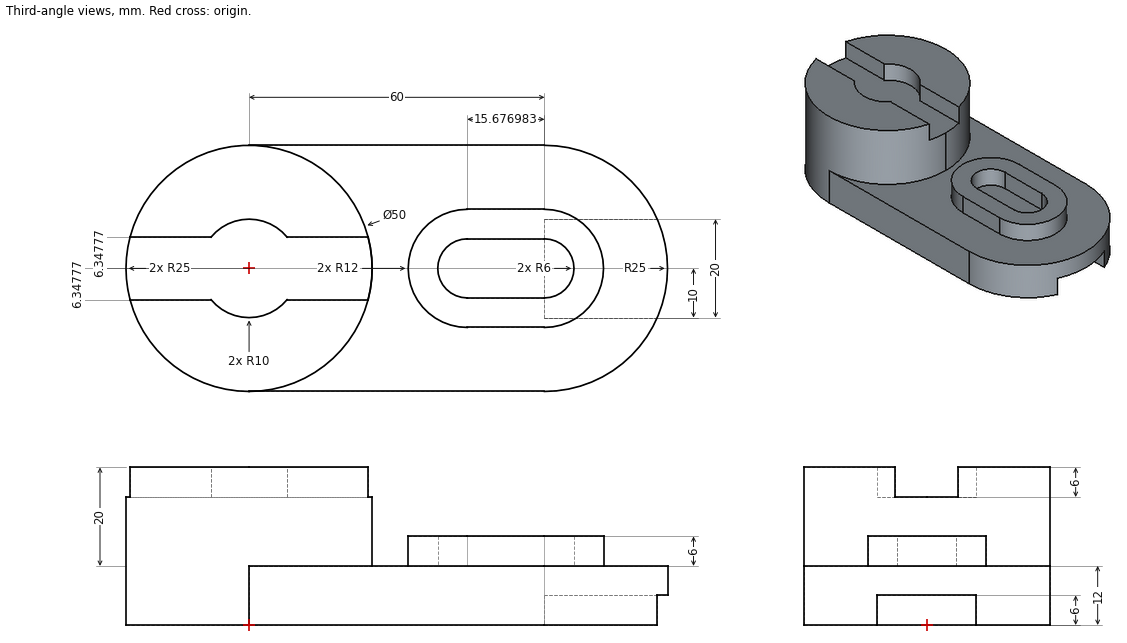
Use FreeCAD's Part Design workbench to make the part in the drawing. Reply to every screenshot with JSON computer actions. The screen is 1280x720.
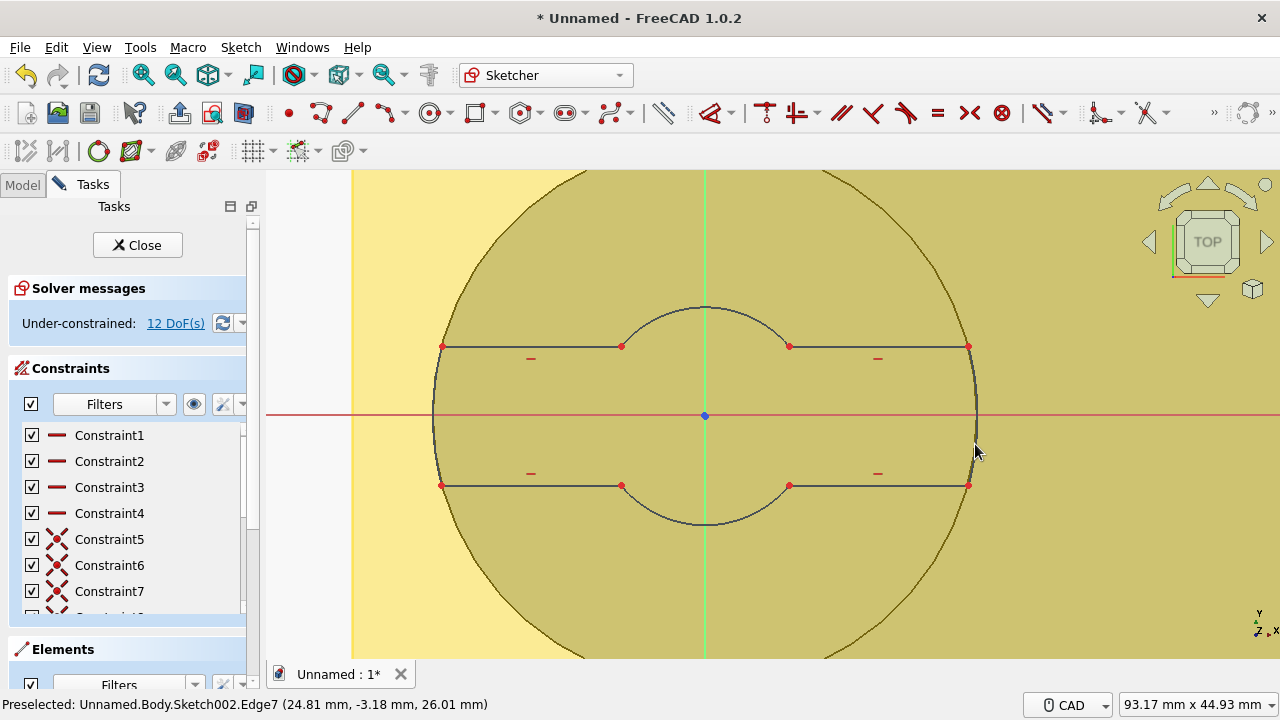
{"action": "left_click", "coordinate": [435, 388]}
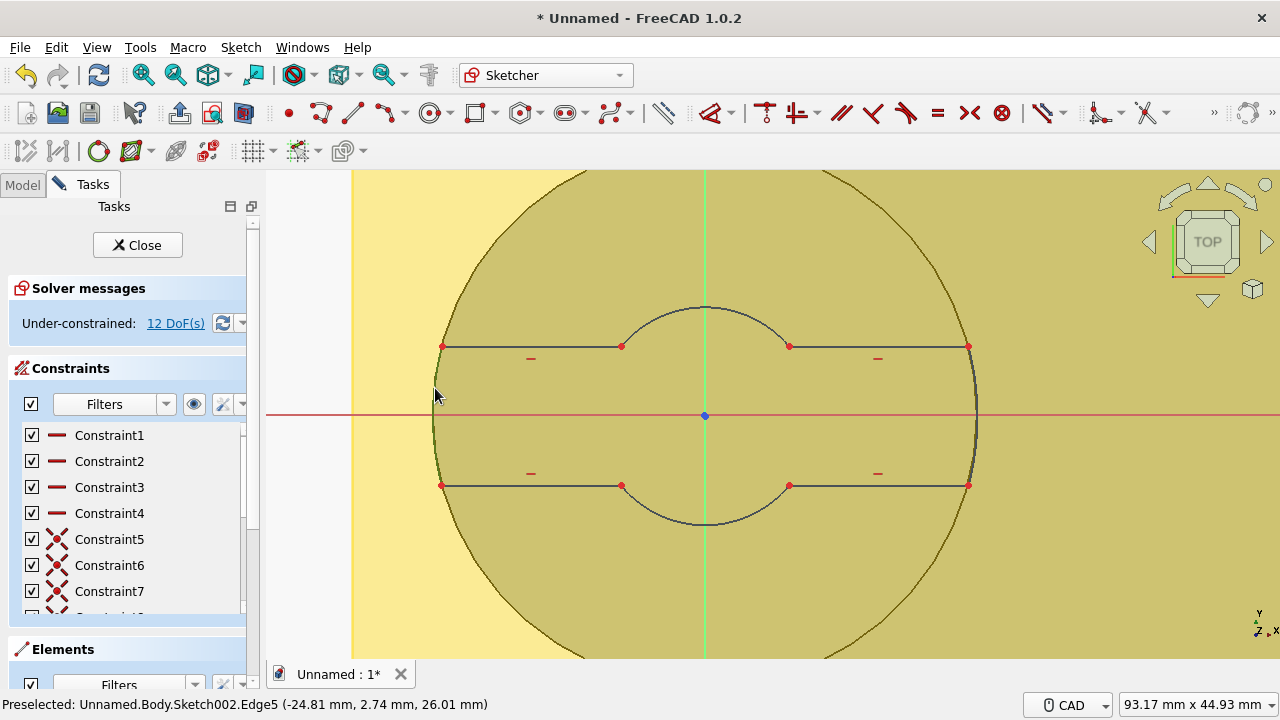
{"action": "left_click", "coordinate": [743, 314]}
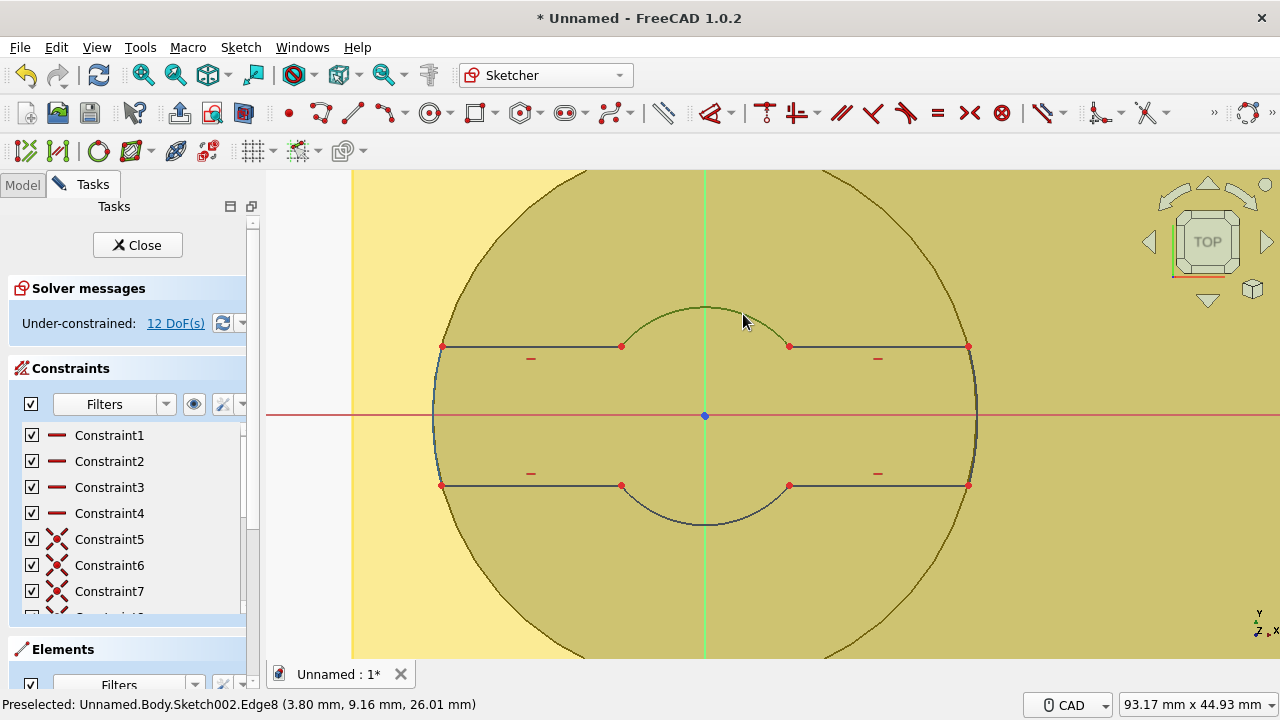
{"action": "left_click", "coordinate": [766, 114]}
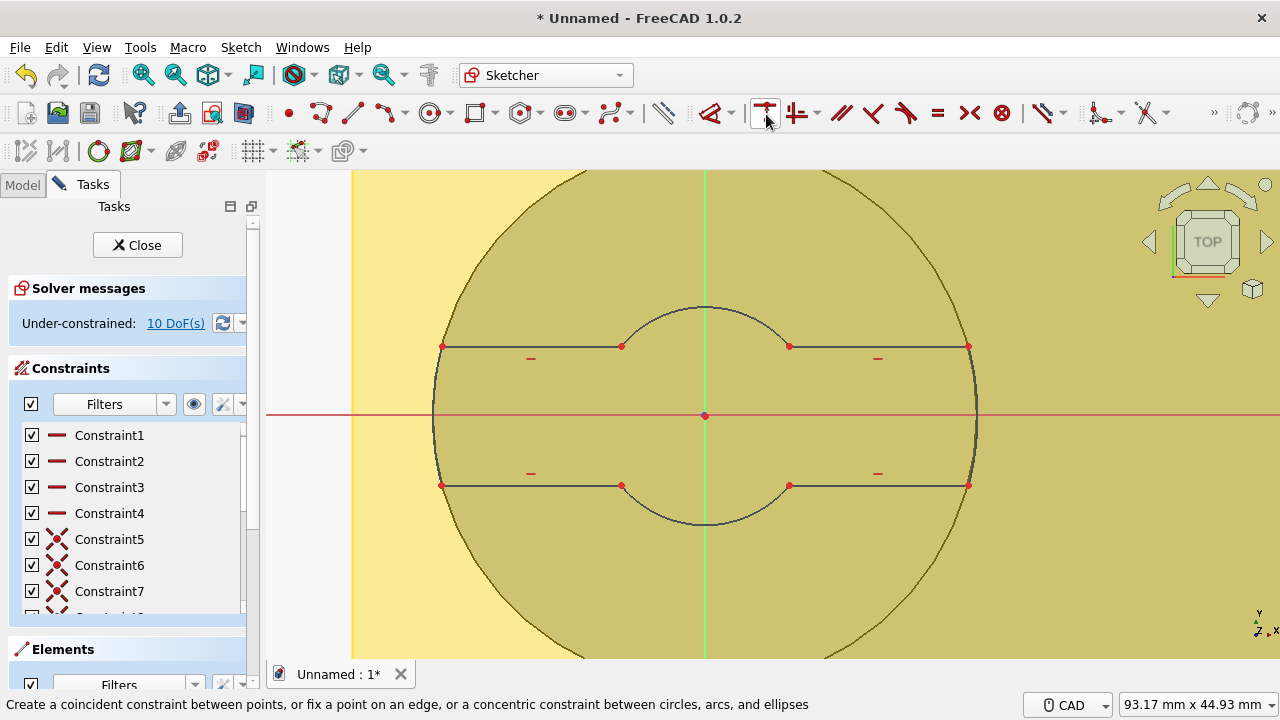
{"action": "left_click_drag", "start_coordinate": [695, 405], "coordinate": [715, 427]}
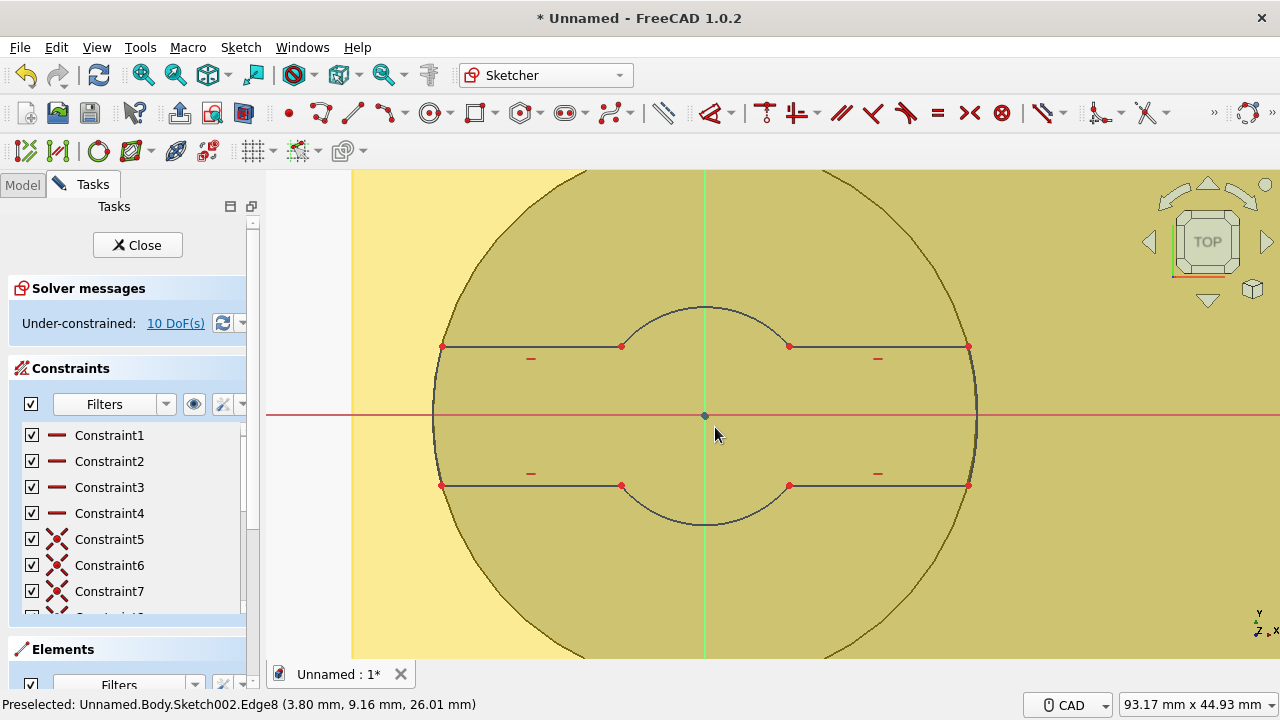
{"action": "key", "text": "c"}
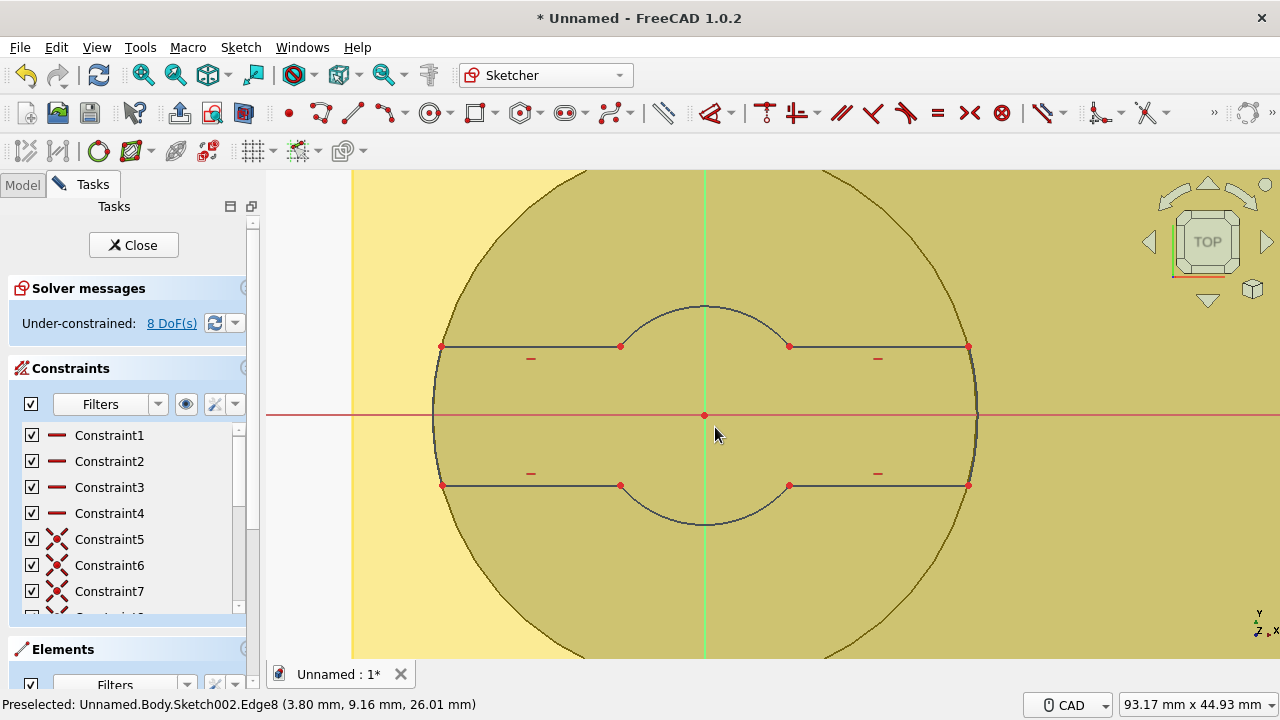
{"action": "left_click", "coordinate": [434, 388]}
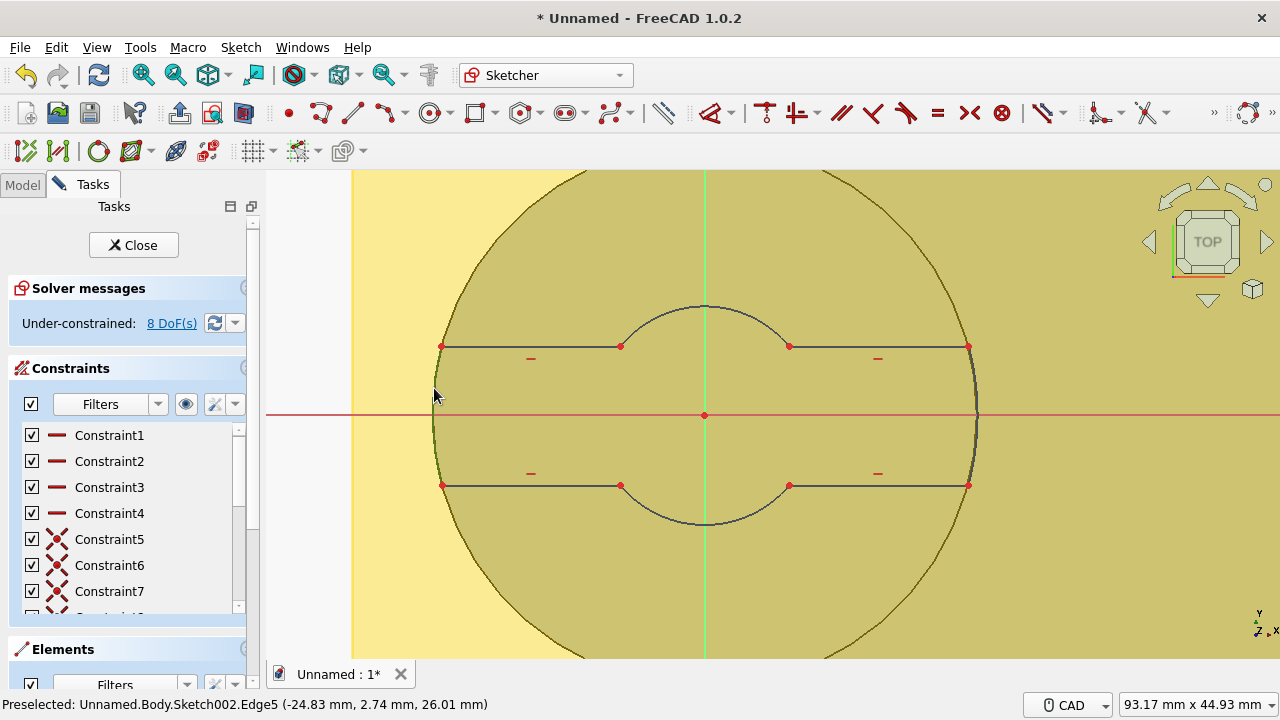
{"action": "left_click", "coordinate": [976, 444]}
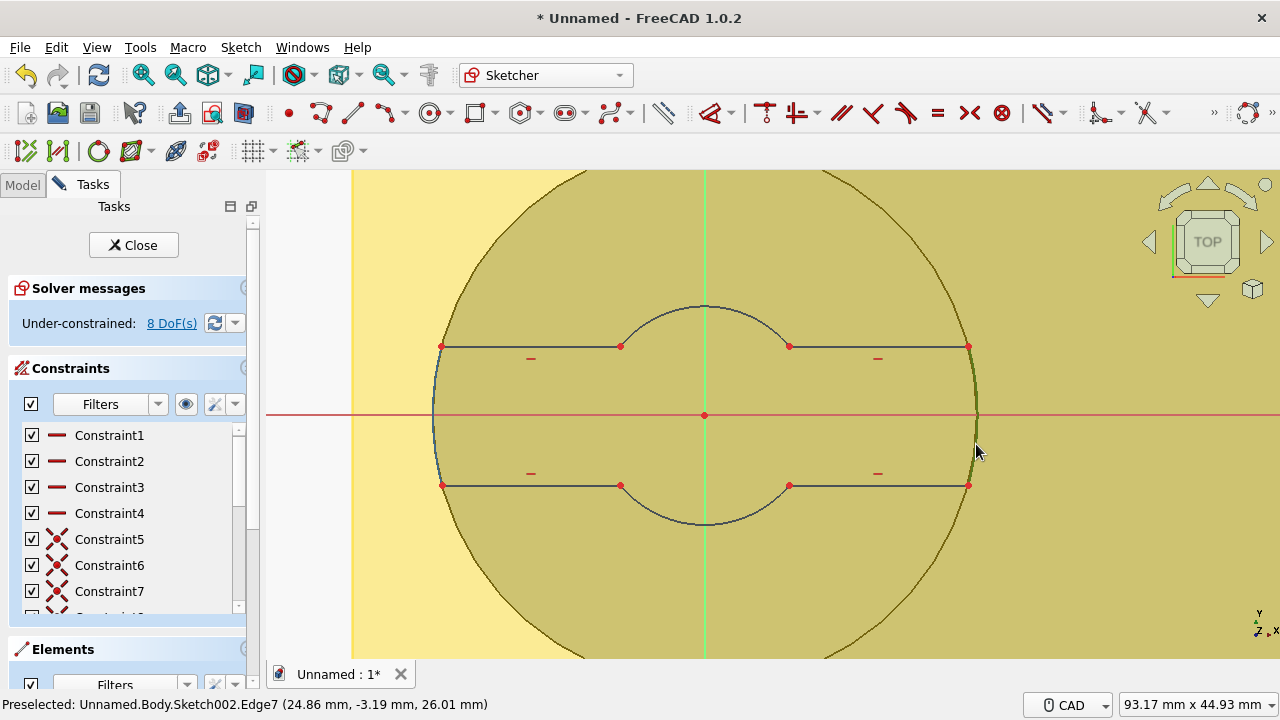
{"action": "left_click", "coordinate": [938, 114]}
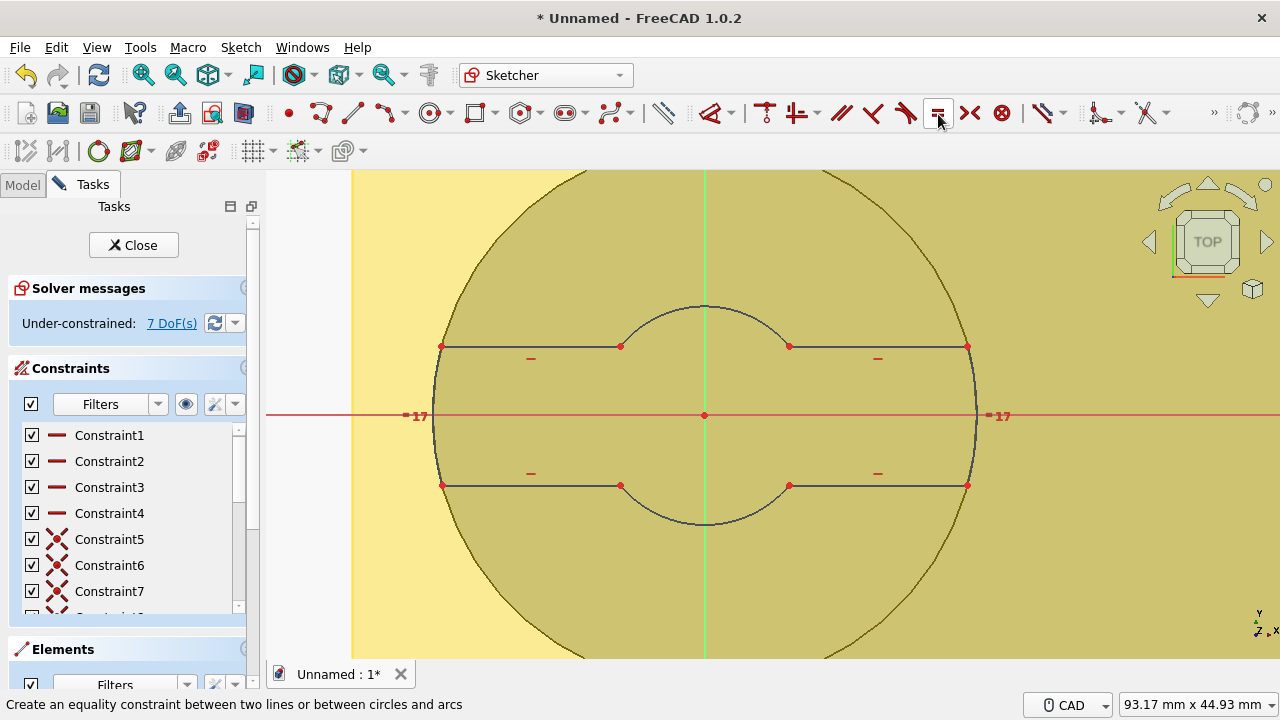
{"action": "left_click", "coordinate": [667, 518]}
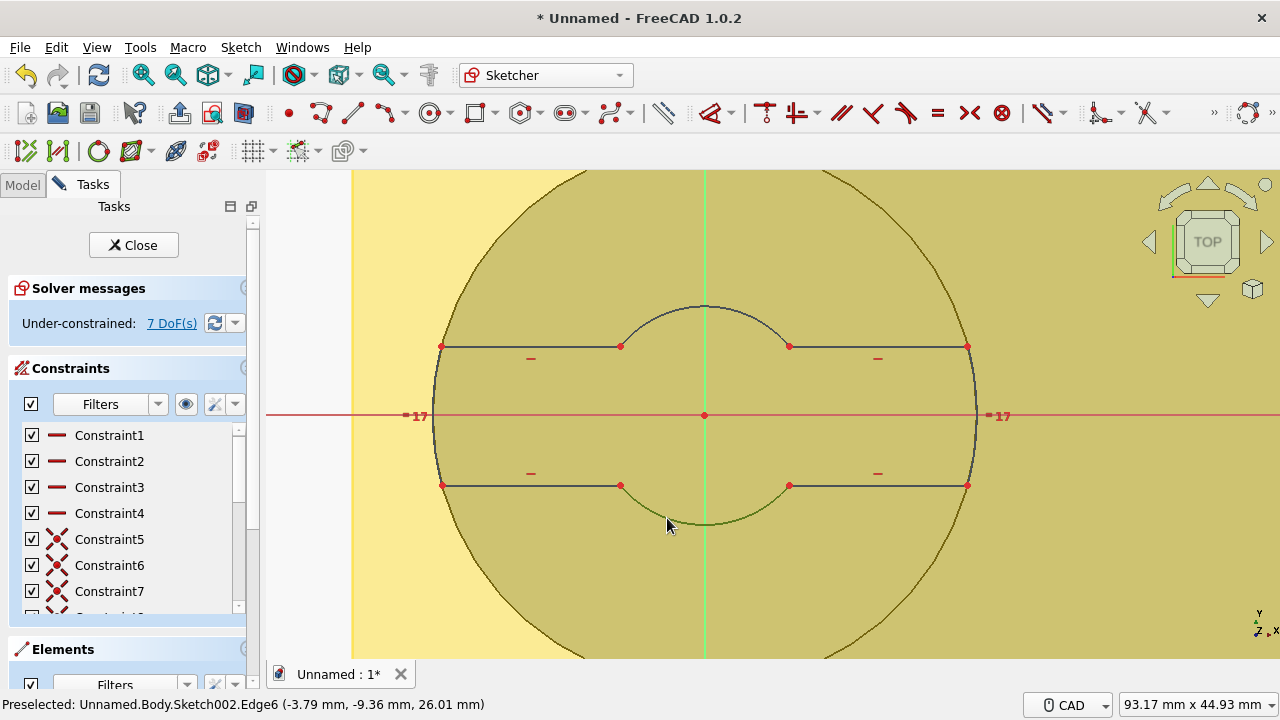
{"action": "left_click", "coordinate": [743, 313]}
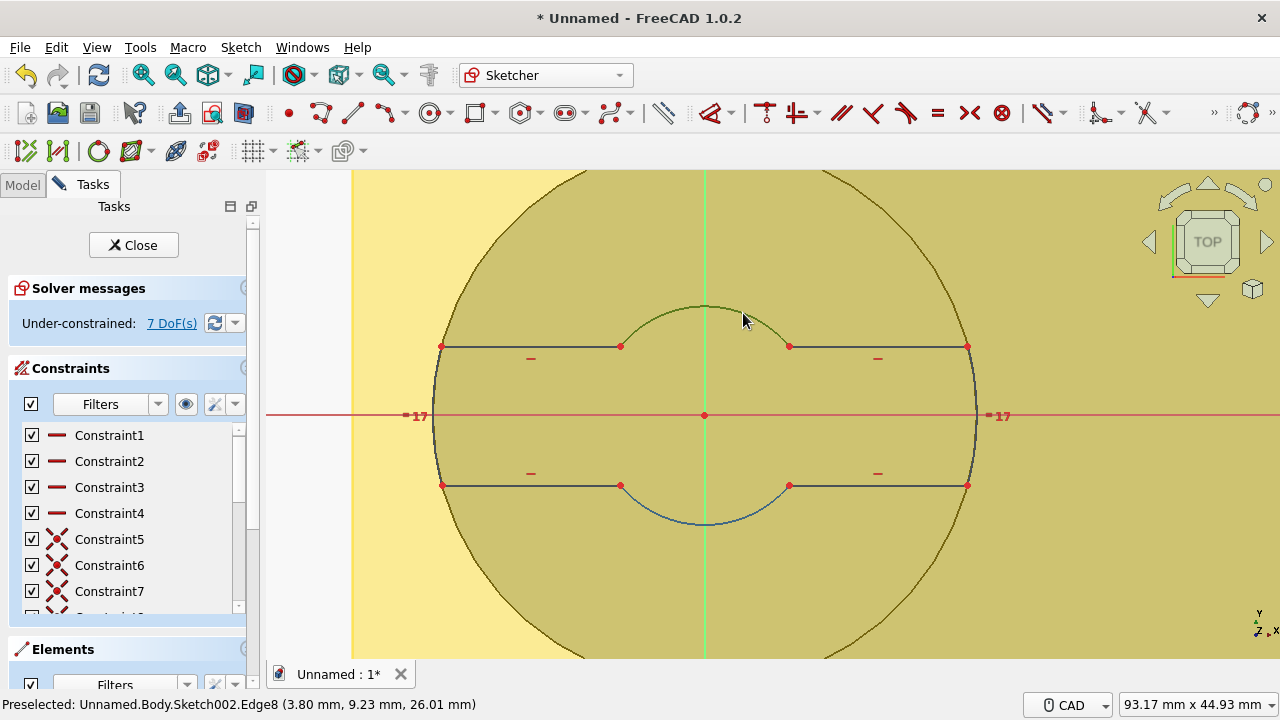
{"action": "key", "text": "e"}